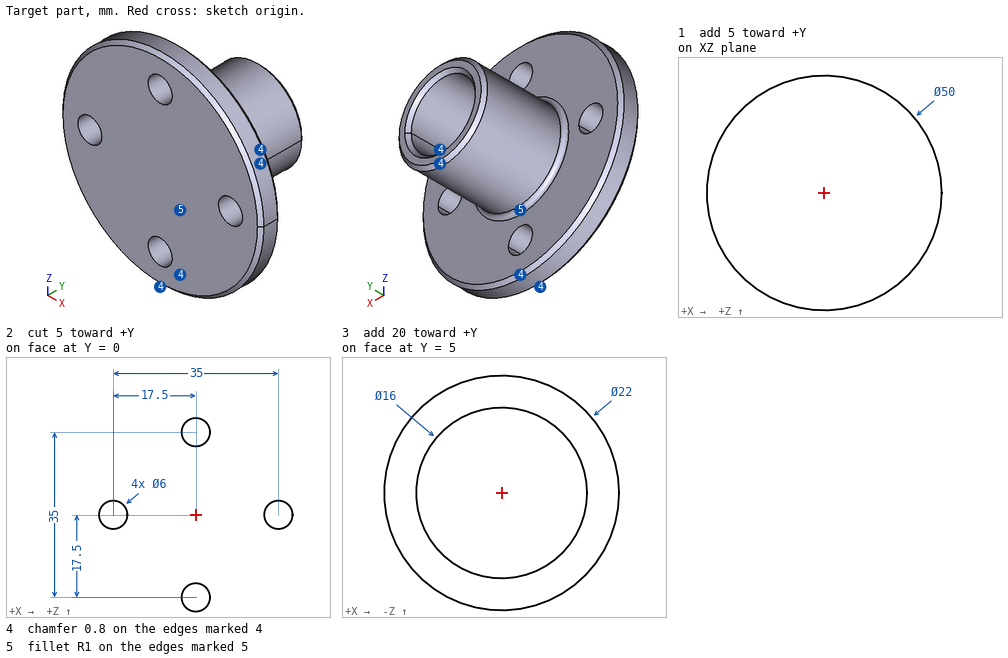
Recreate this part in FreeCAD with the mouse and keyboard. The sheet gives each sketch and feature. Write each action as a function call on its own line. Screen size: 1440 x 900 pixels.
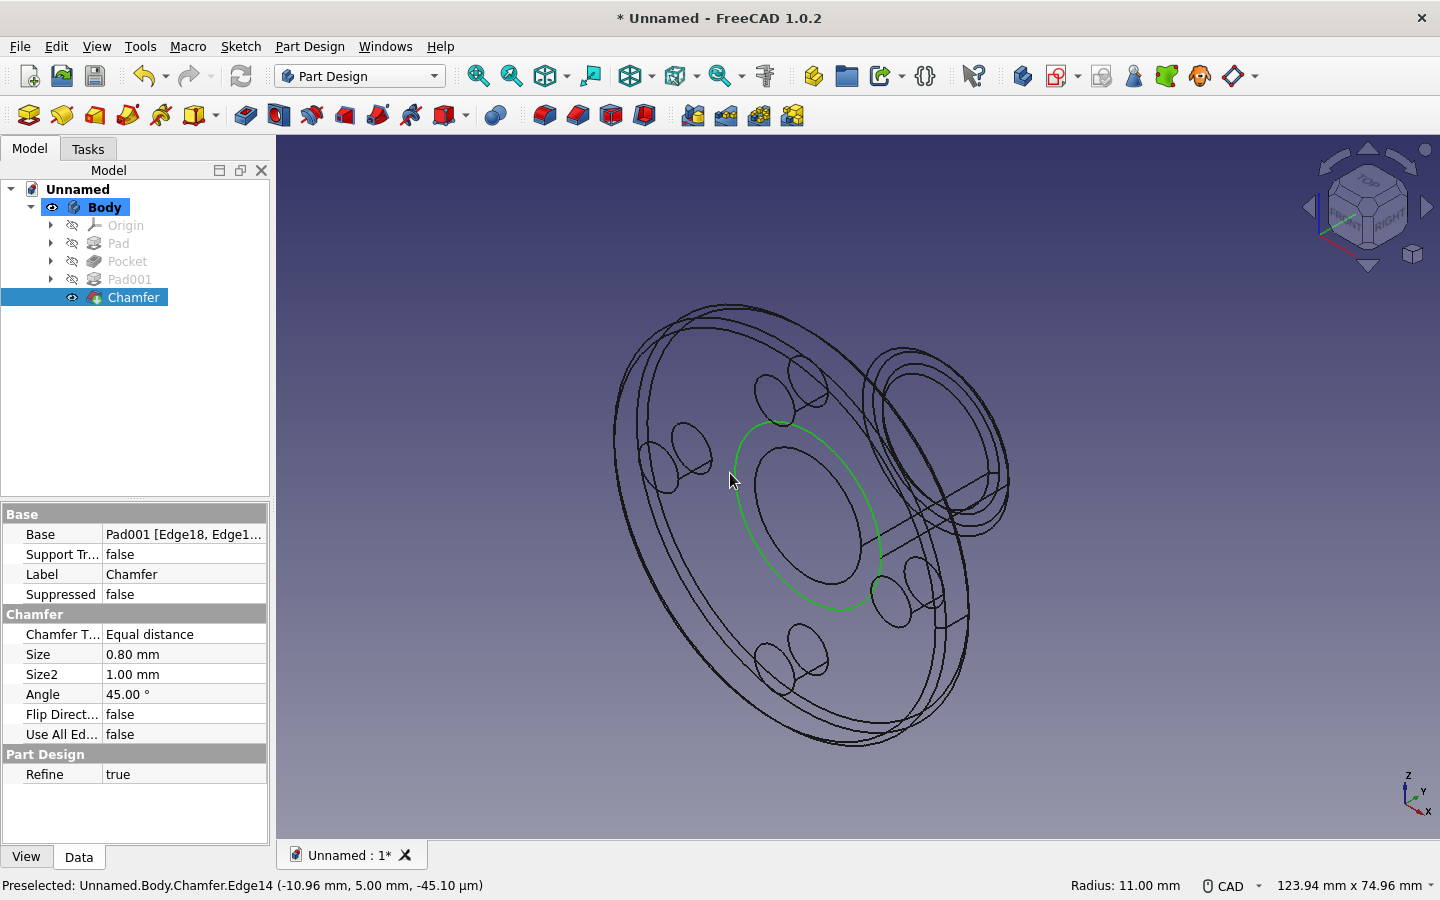
key(v)
key(1)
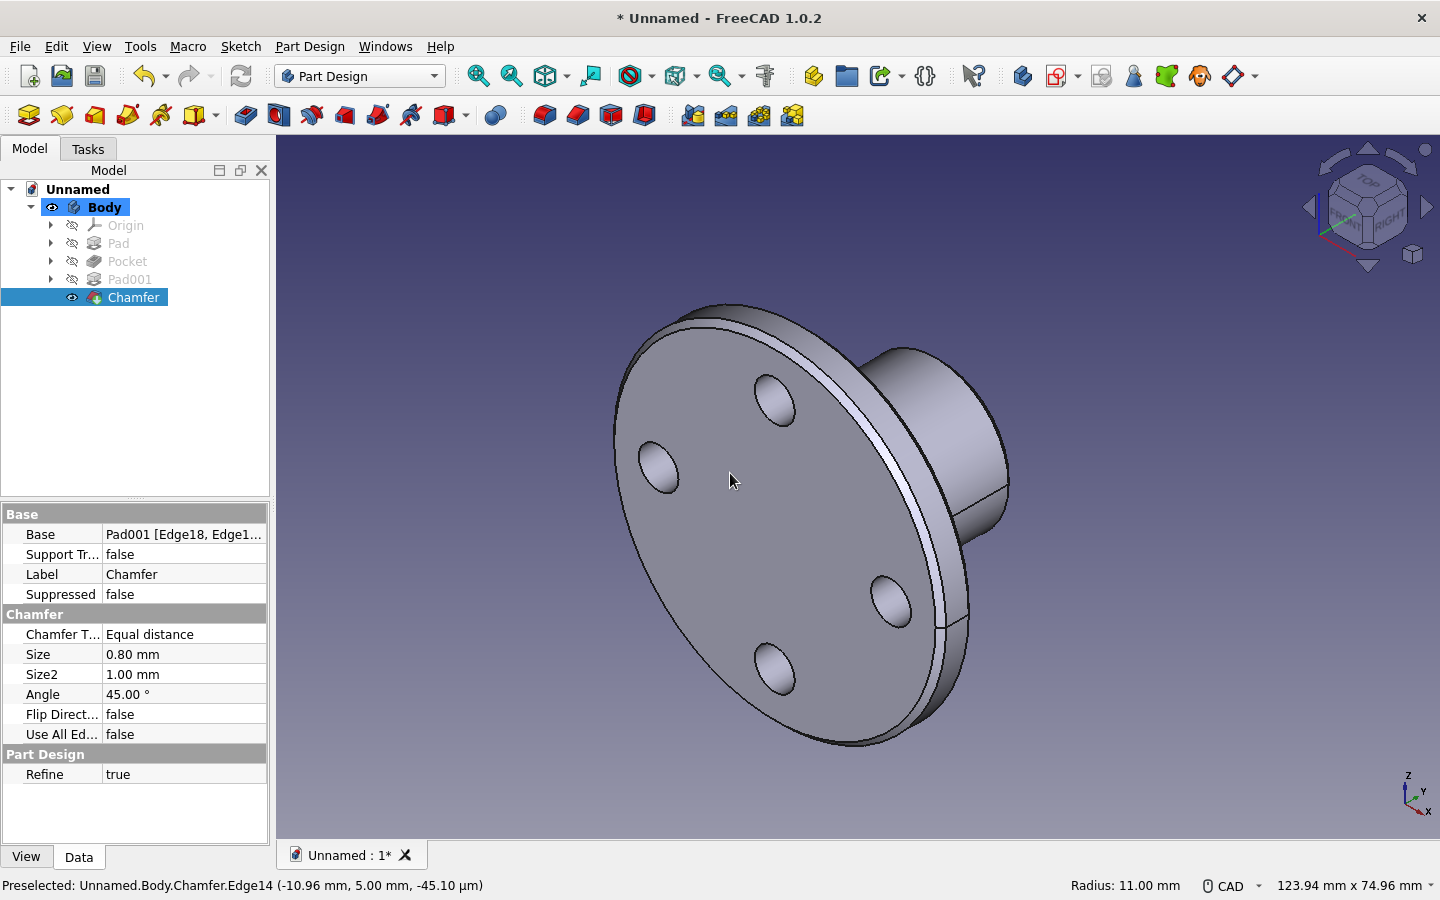
click(545, 116)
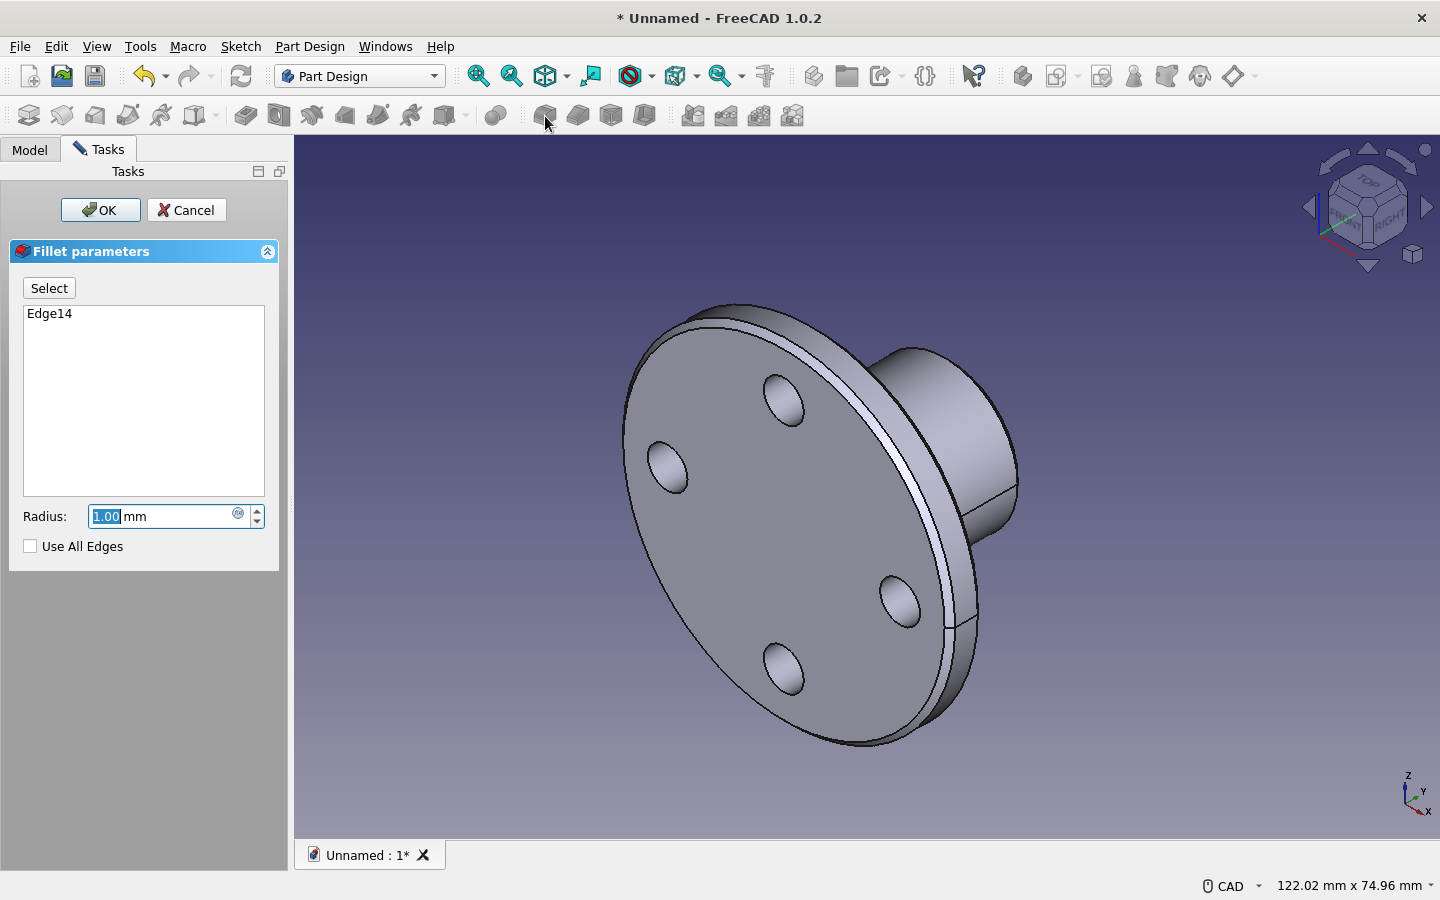
text(1)
key(Tab)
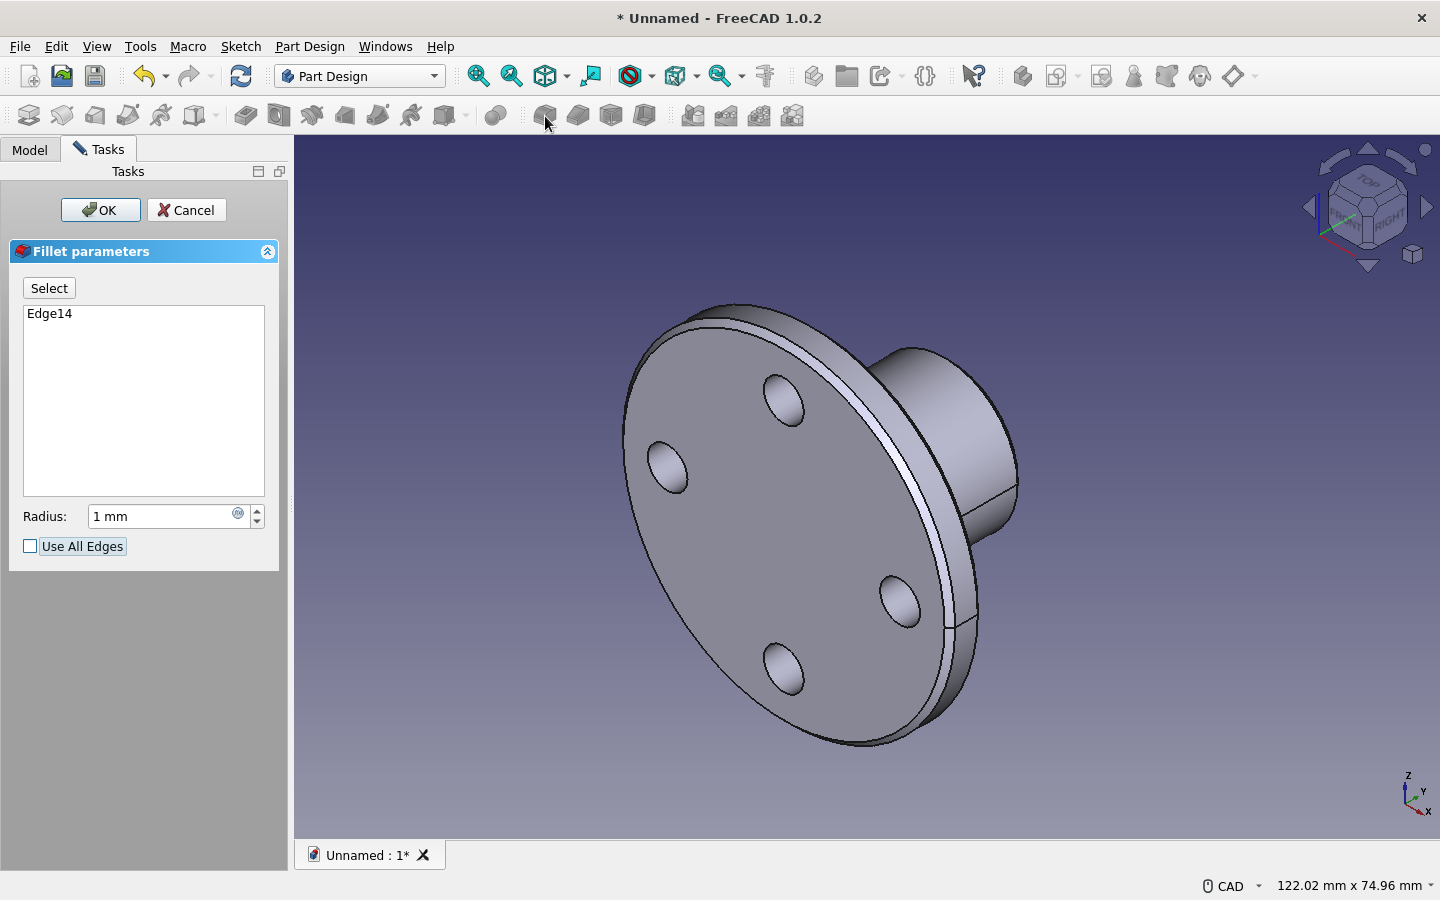
click(101, 210)